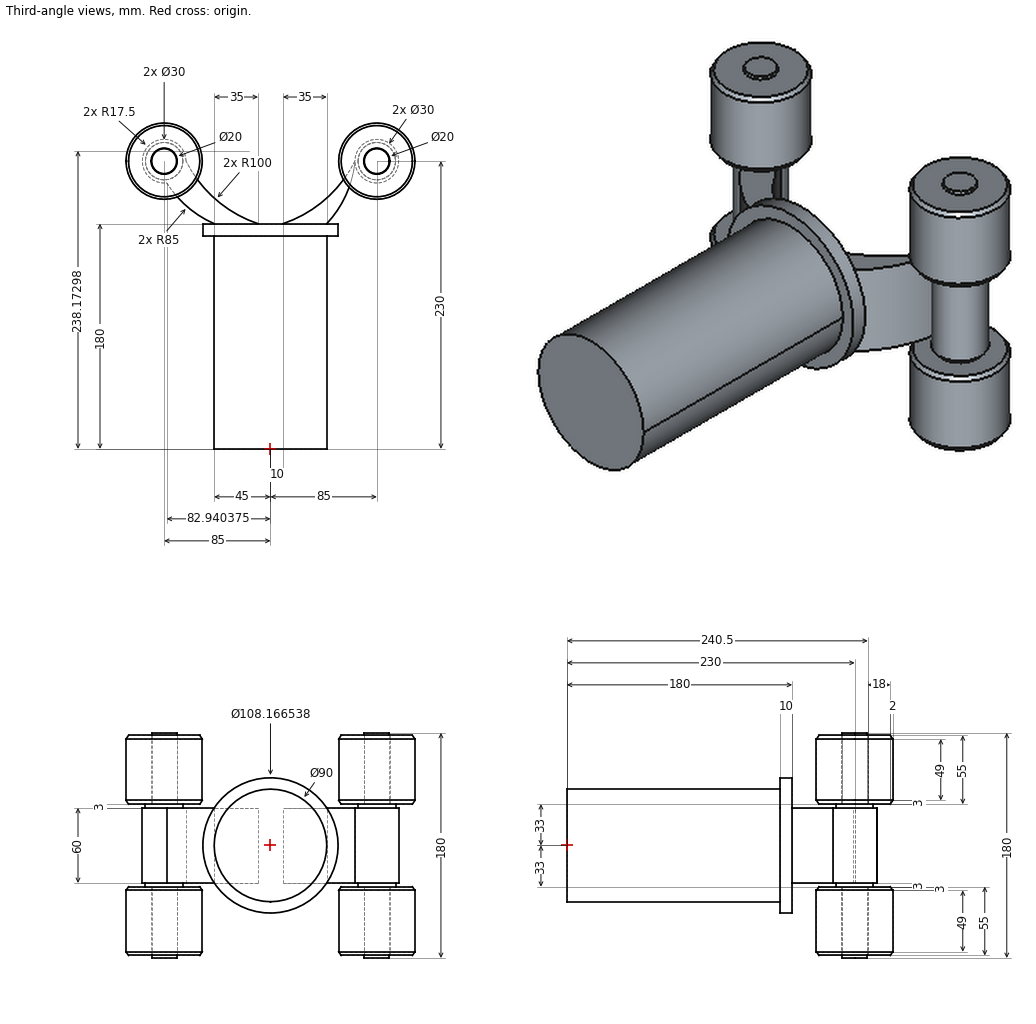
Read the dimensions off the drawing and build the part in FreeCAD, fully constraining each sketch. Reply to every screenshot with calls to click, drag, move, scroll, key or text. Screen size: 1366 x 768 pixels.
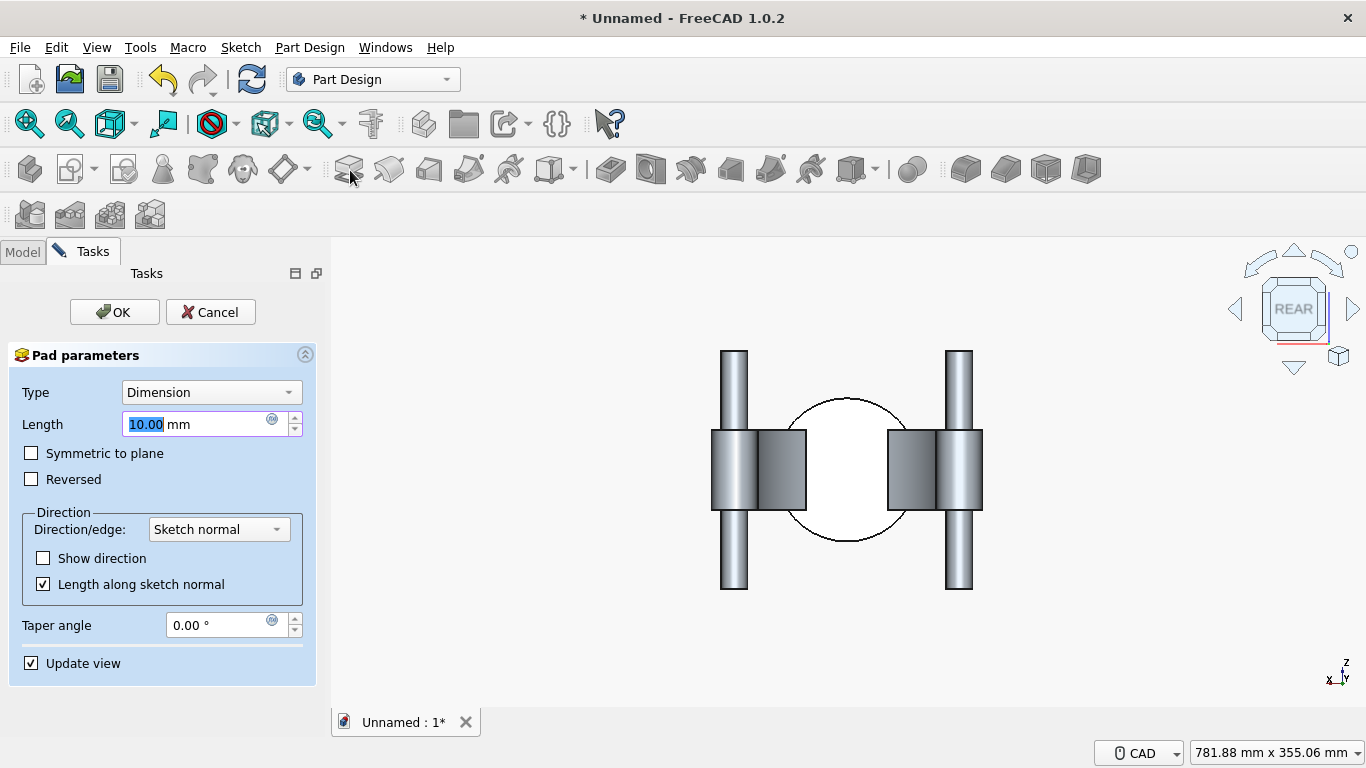
text(10)
key(Tab)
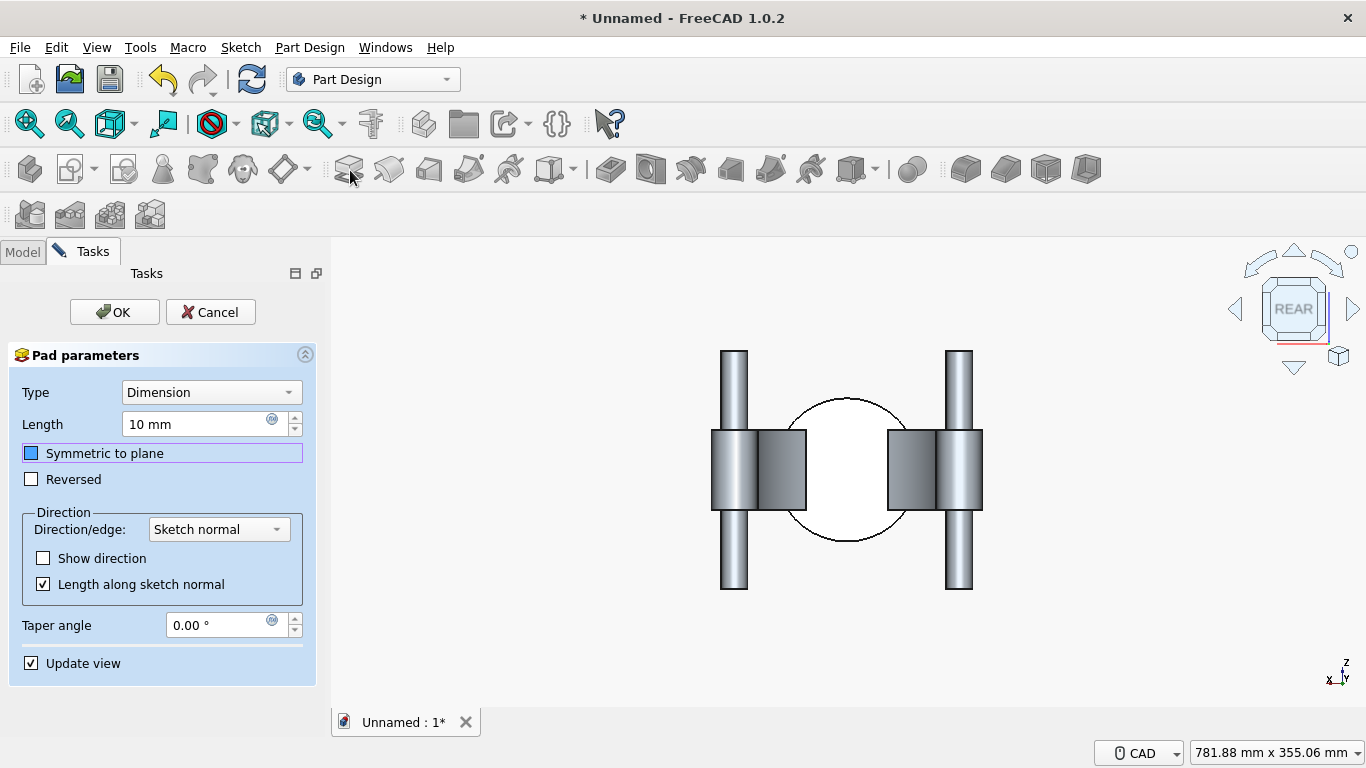
click(30, 479)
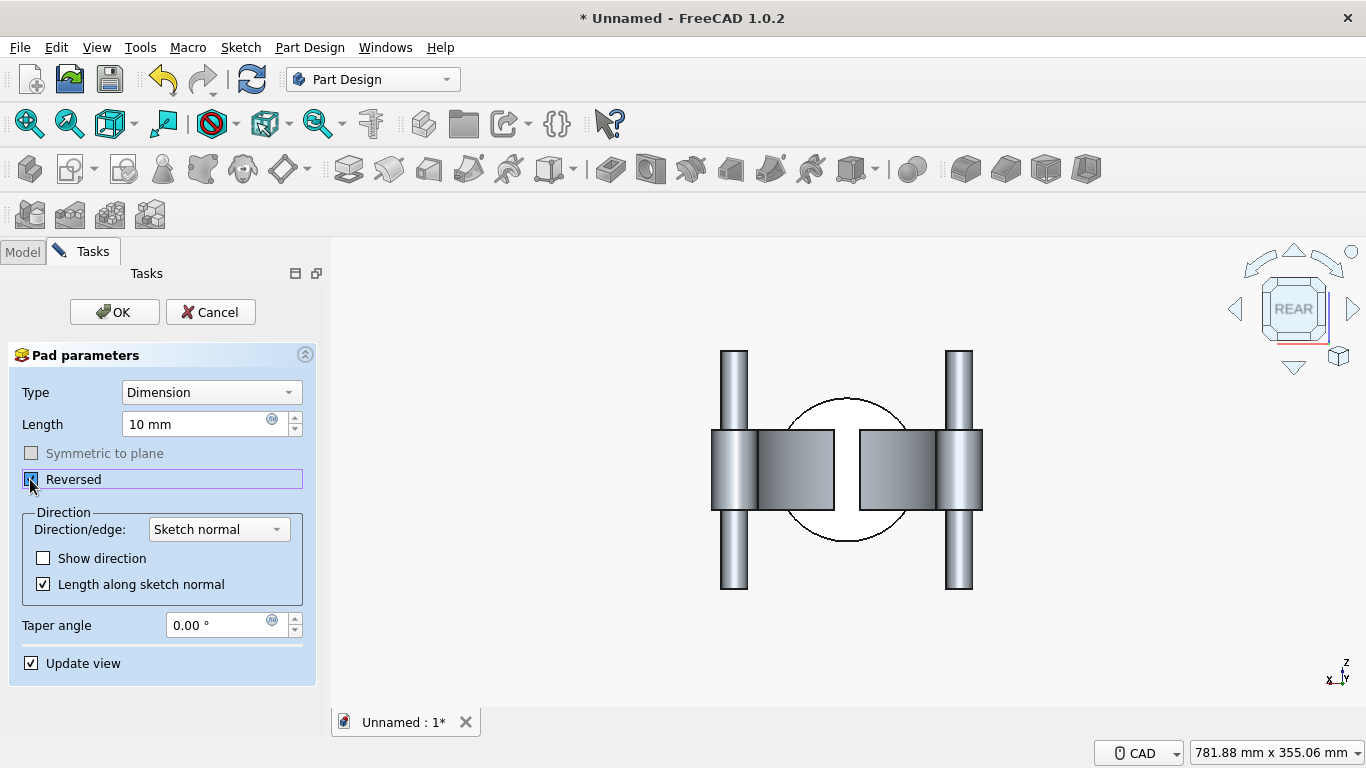
click(115, 312)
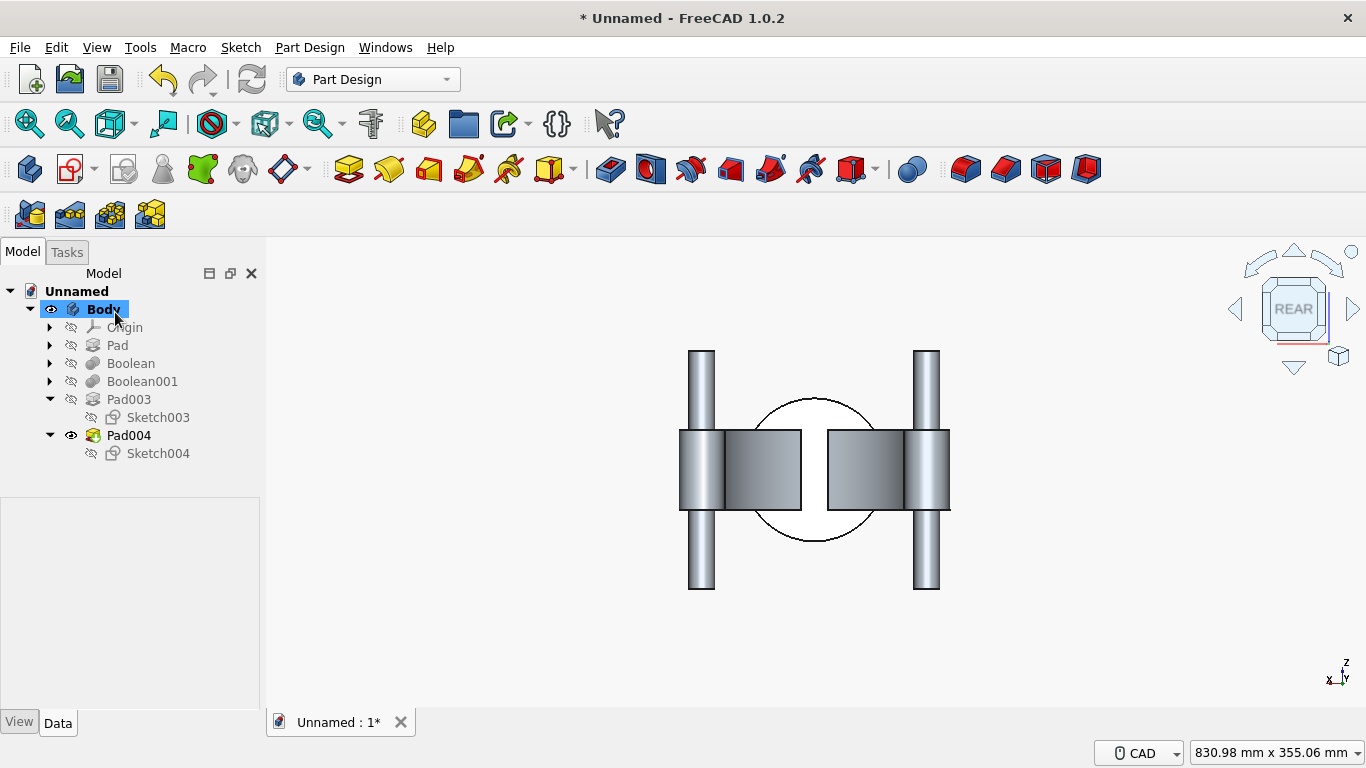
key(0)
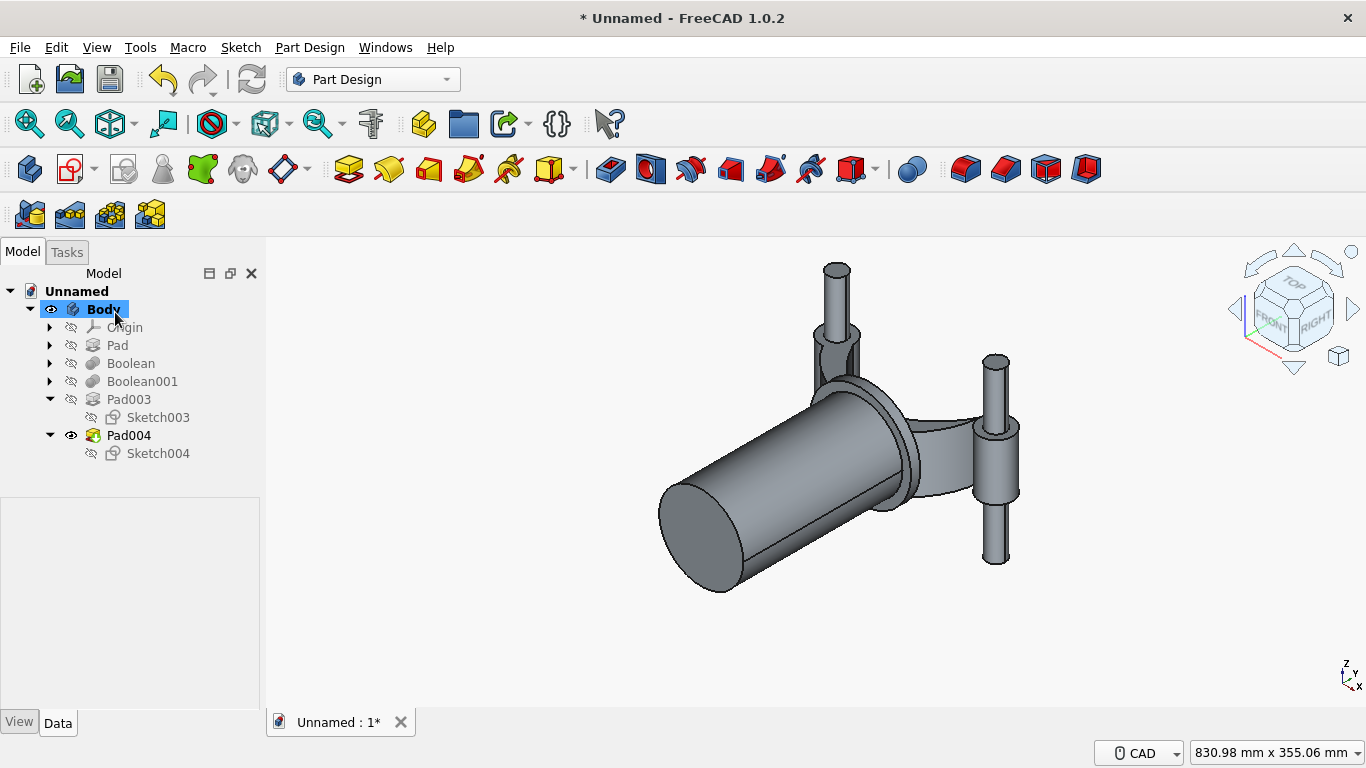
click(836, 351)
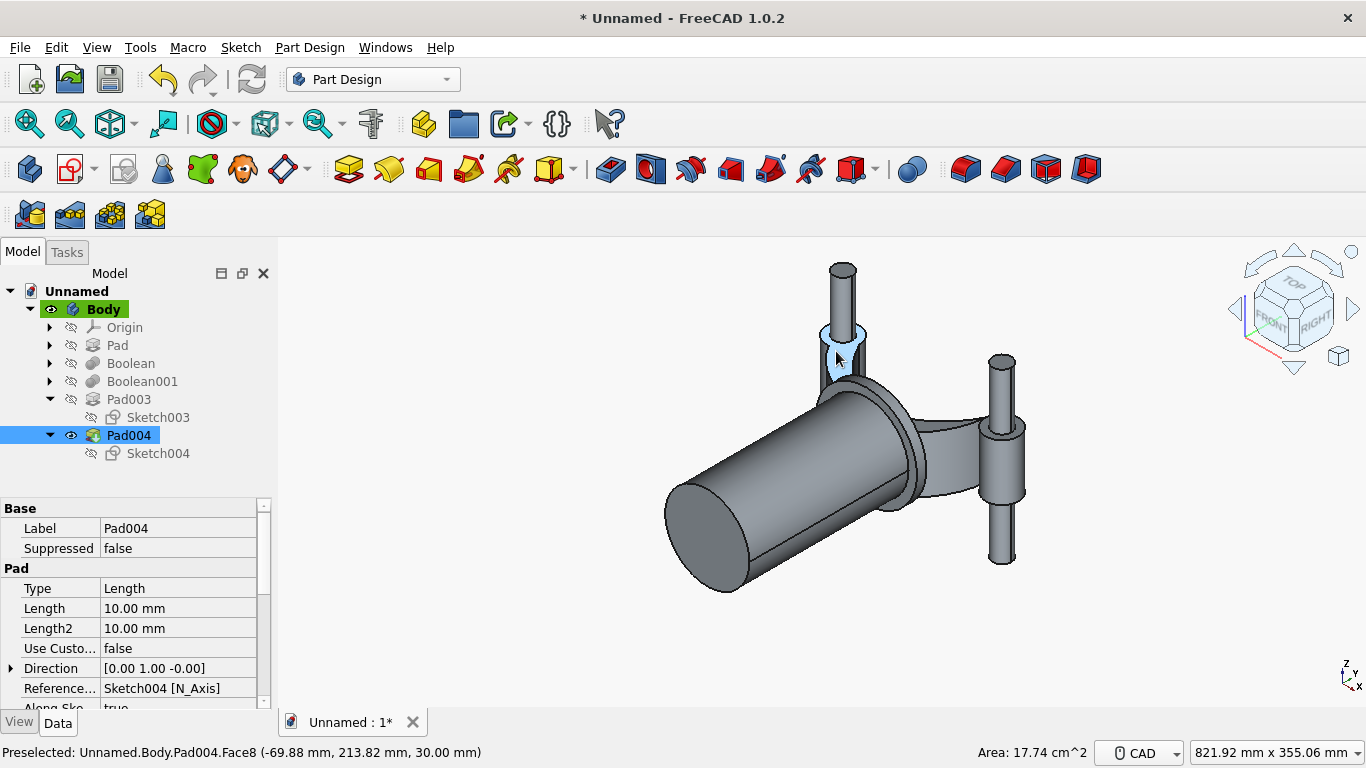
click(70, 170)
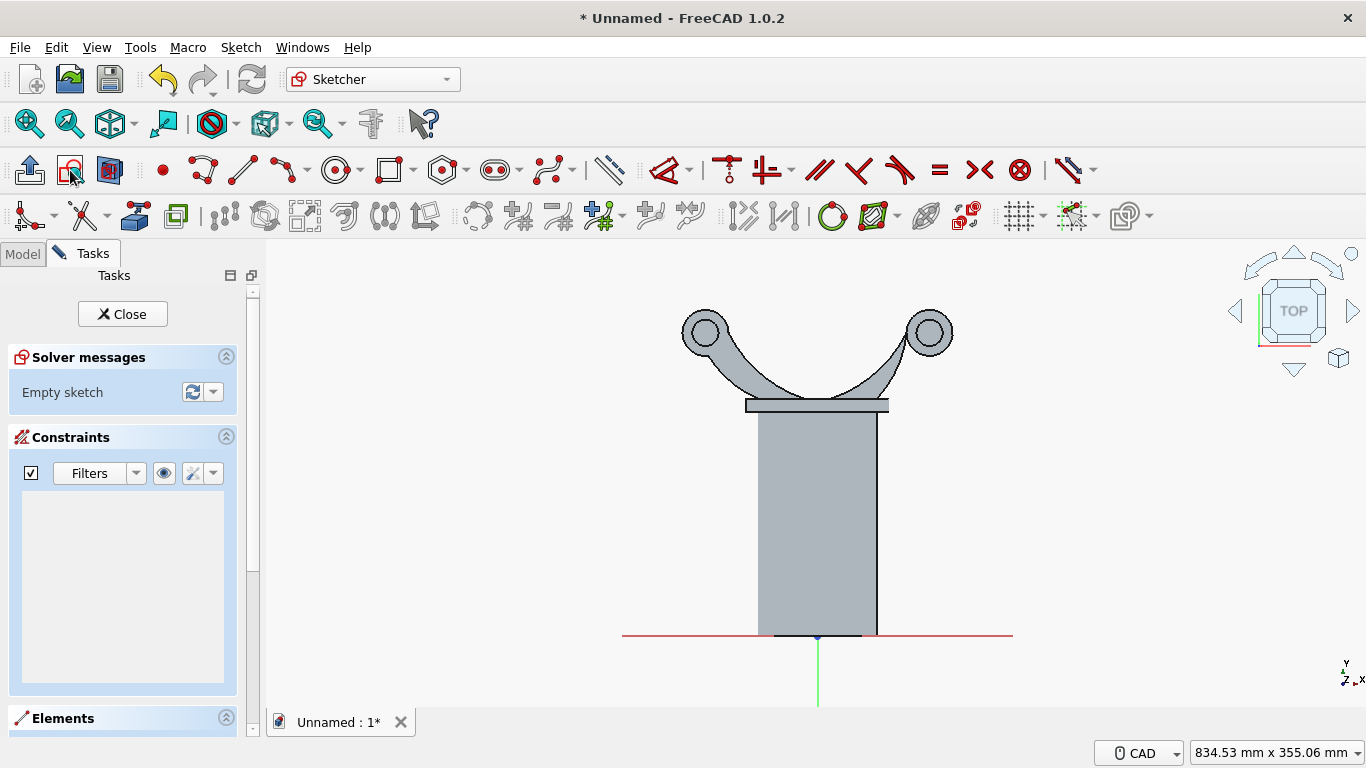
click(336, 170)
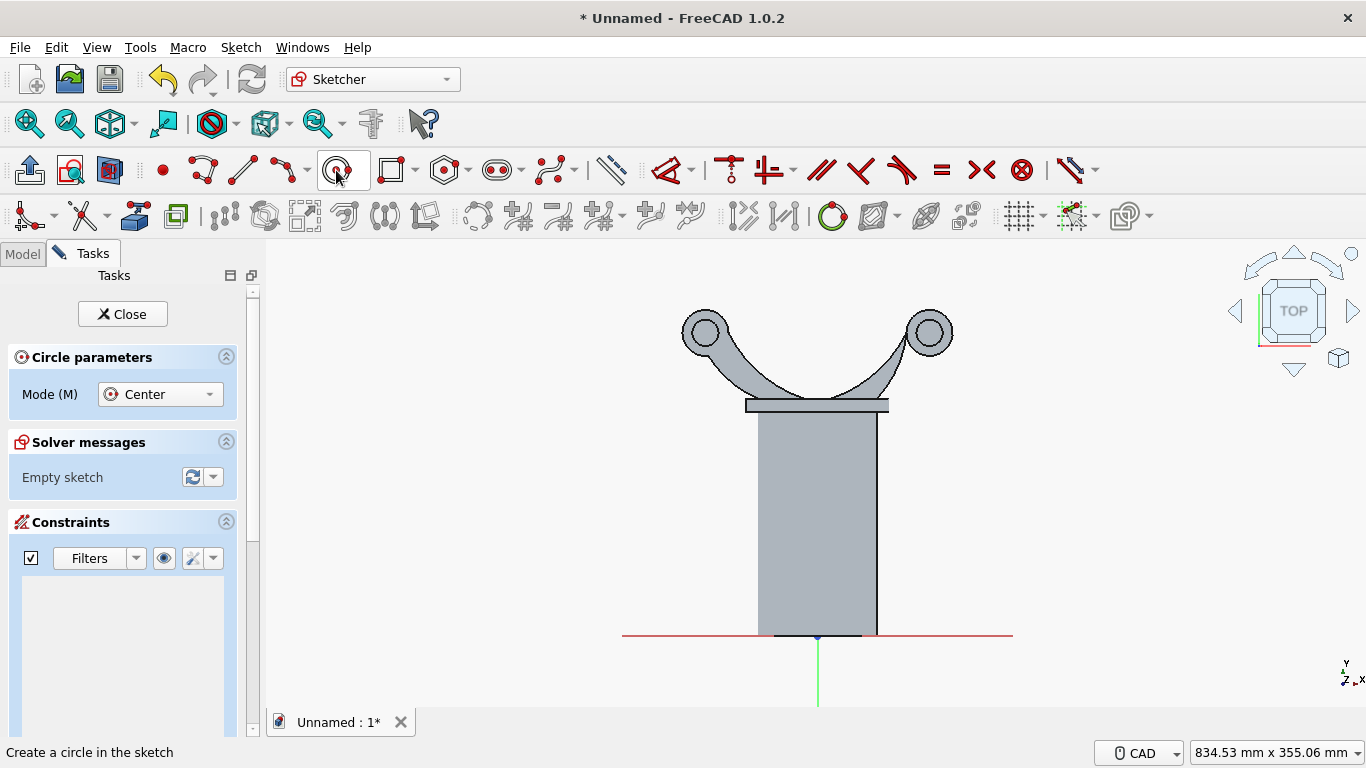
click(705, 333)
click(719, 319)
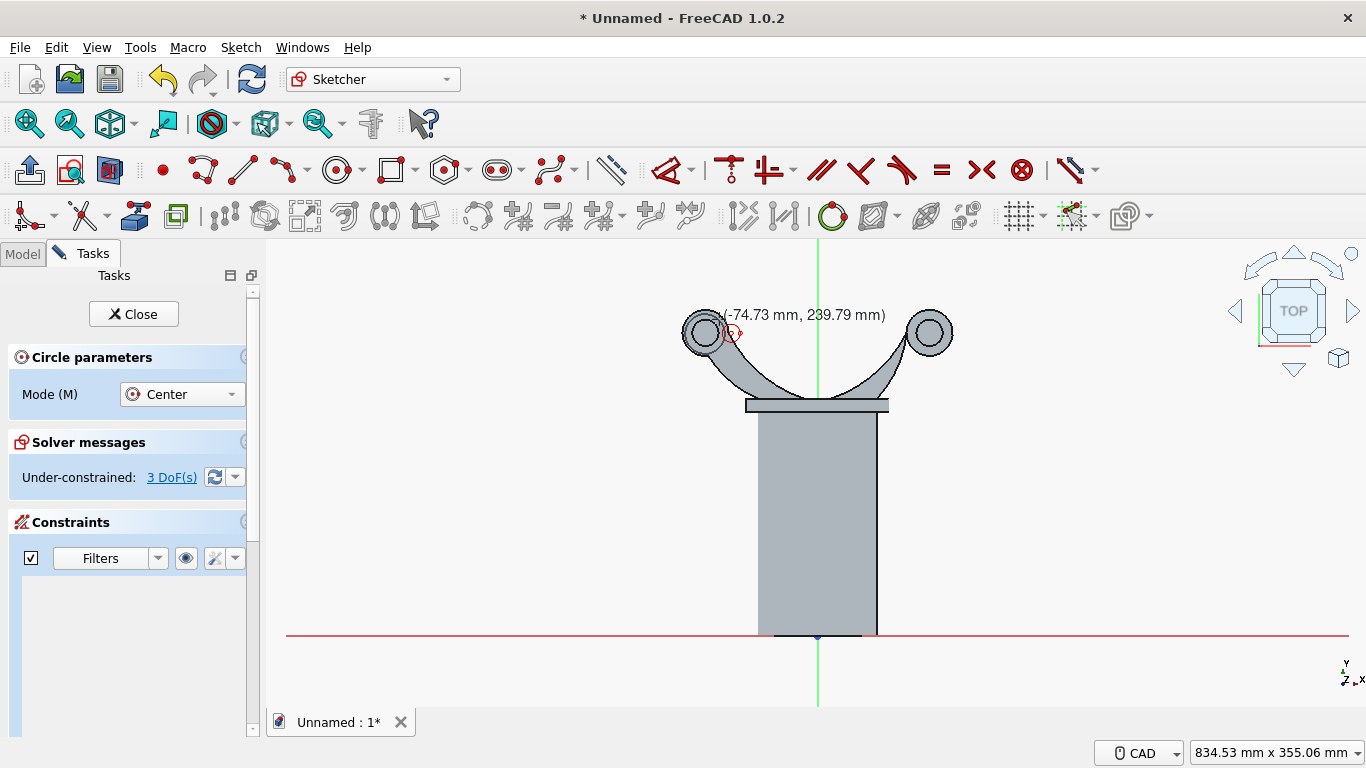
click(930, 333)
click(944, 319)
key(Escape)